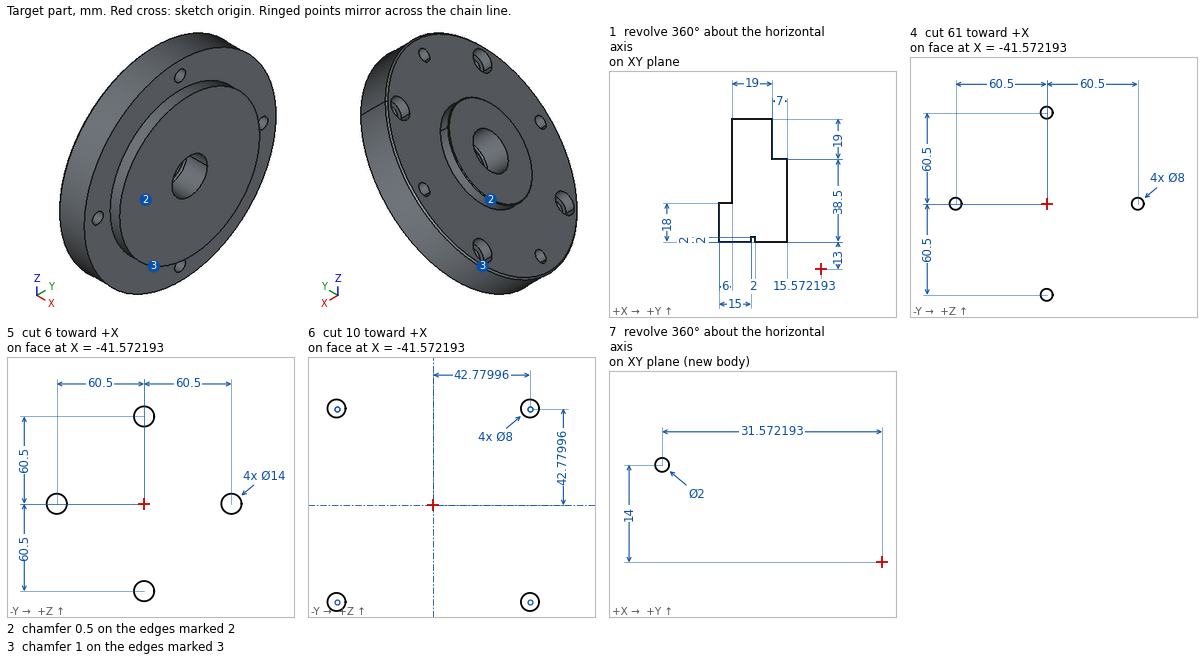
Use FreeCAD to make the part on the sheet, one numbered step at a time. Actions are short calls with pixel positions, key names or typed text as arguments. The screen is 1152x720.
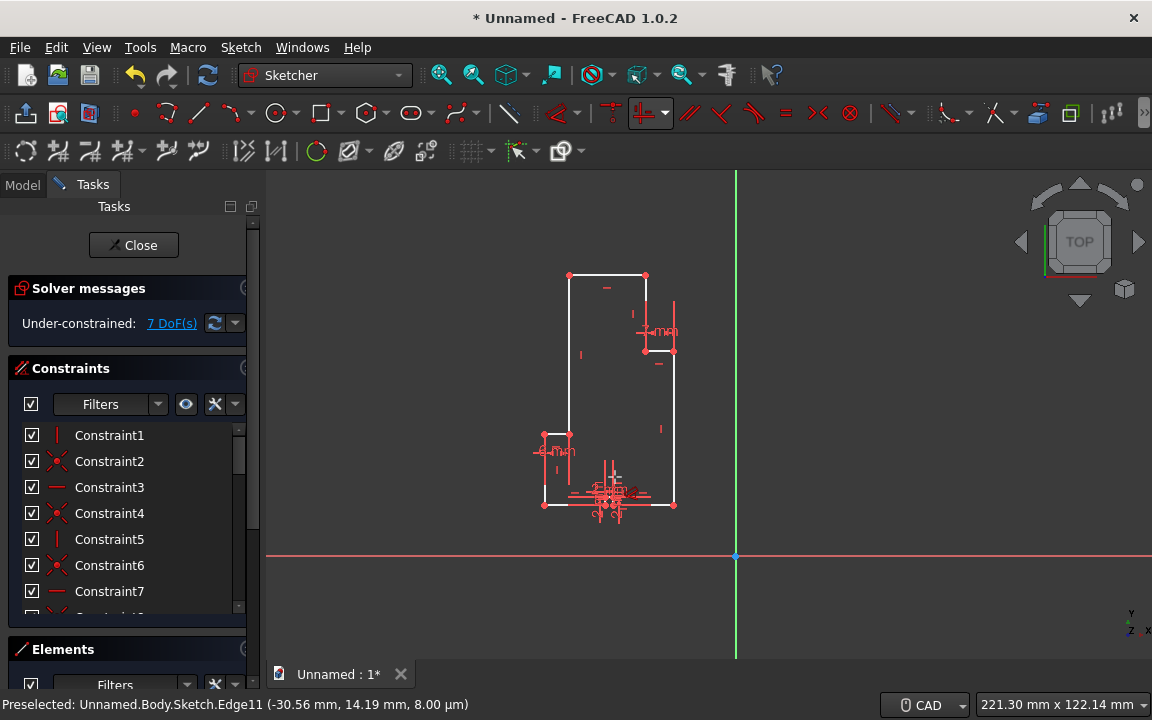
click(646, 328)
click(680, 296)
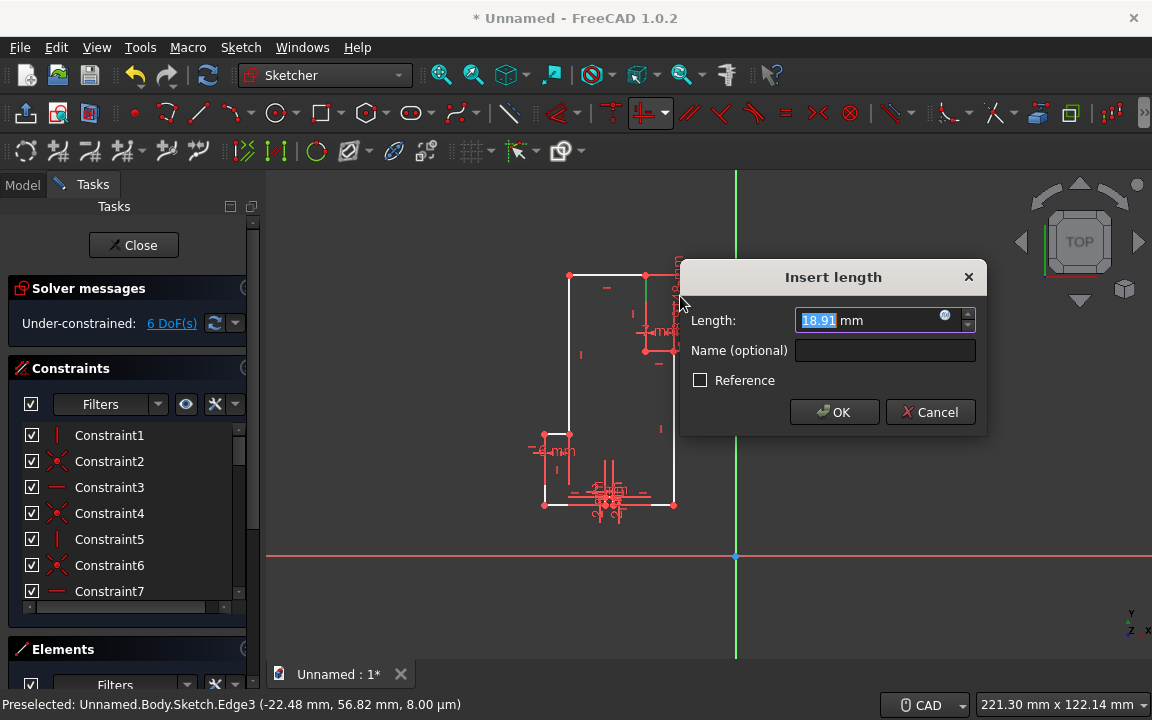
text(19)
key(Return)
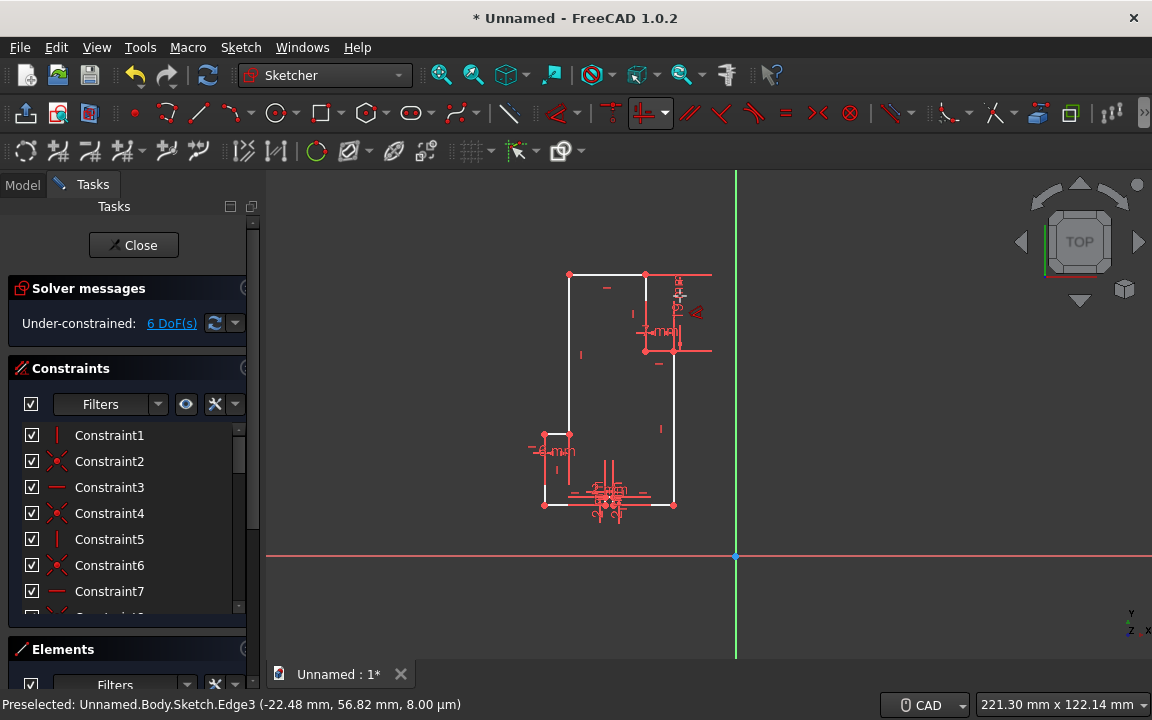
click(623, 275)
click(607, 241)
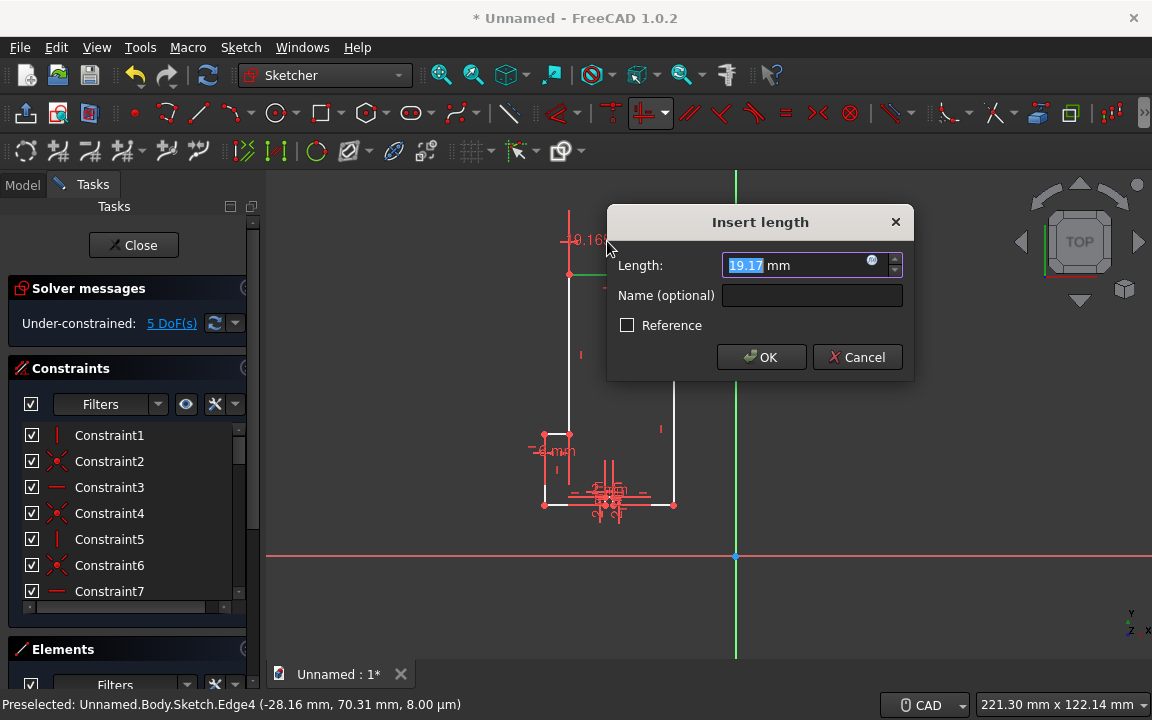
text(19)
key(Return)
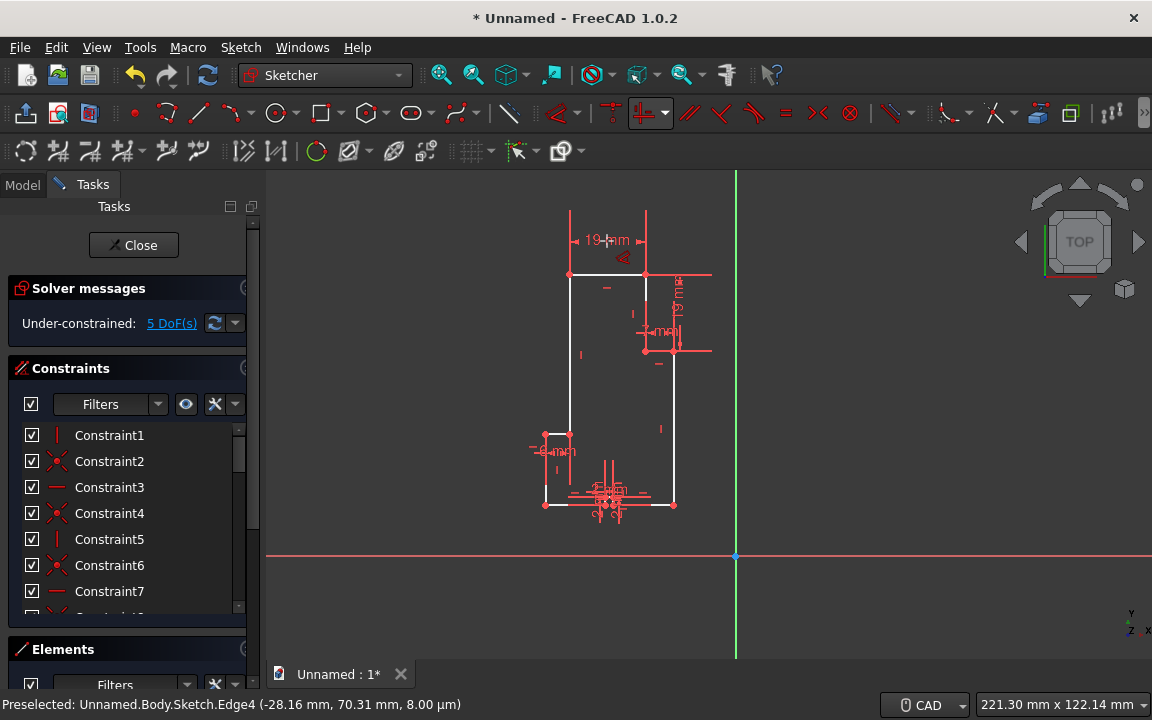
click(546, 455)
click(512, 486)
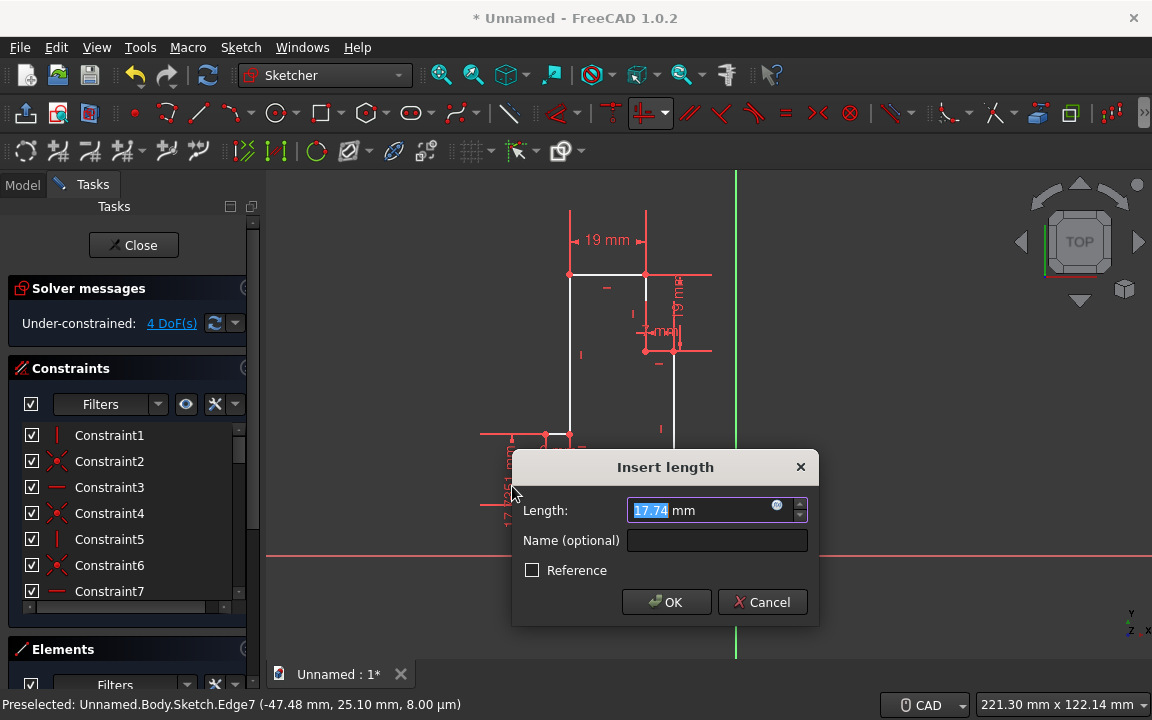
text(18)
key(Return)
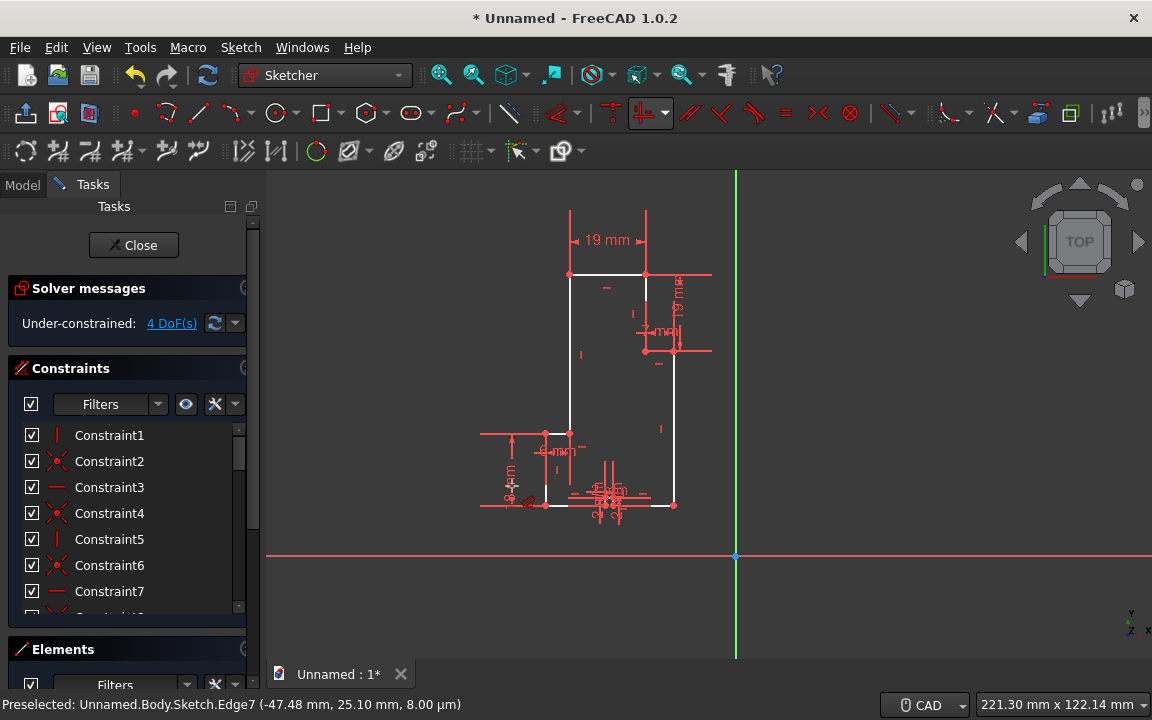
click(564, 506)
click(576, 540)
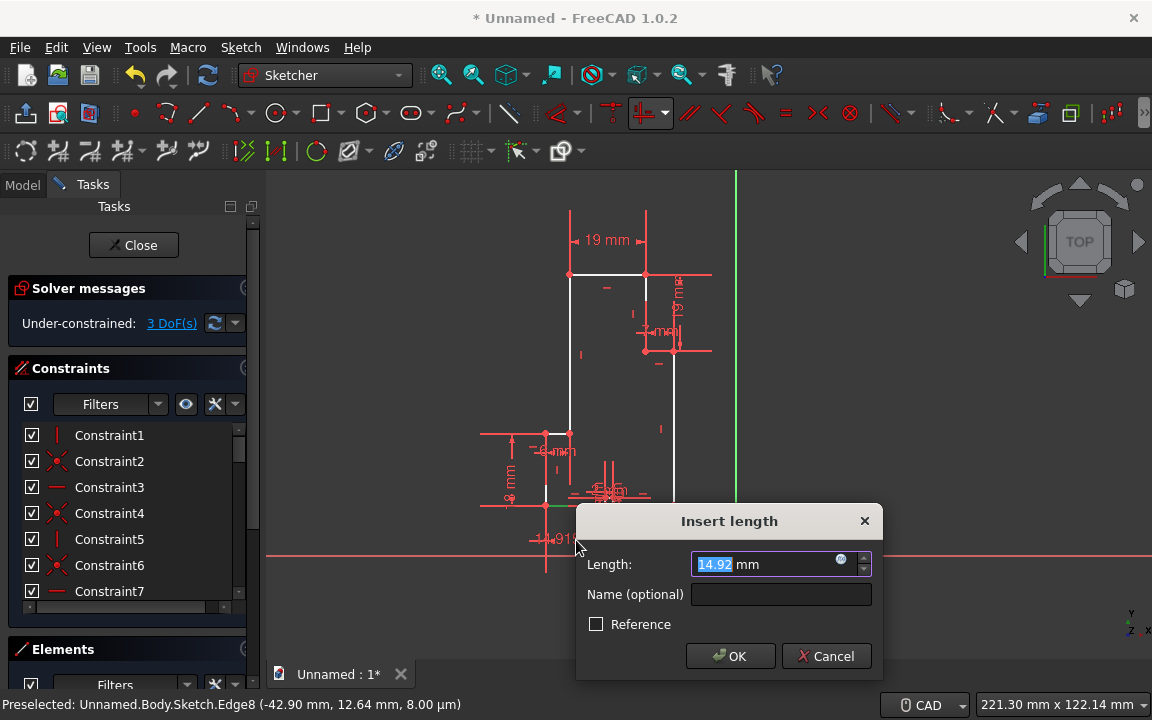
text(15)
key(Return)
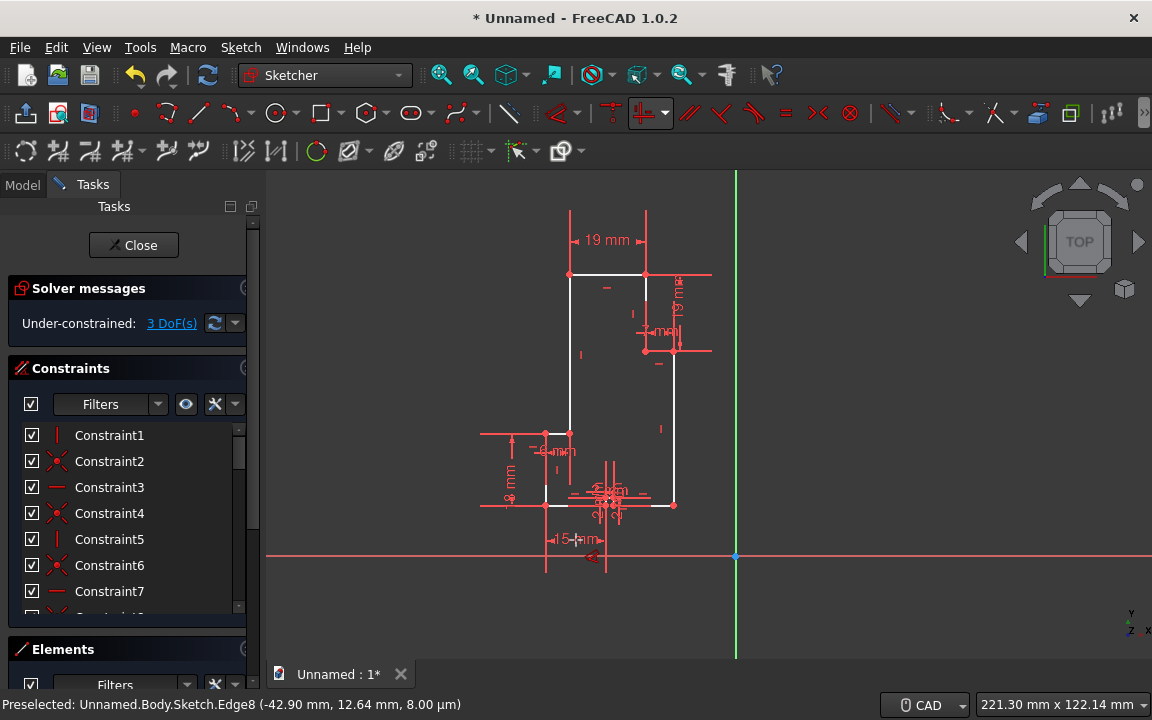
click(674, 506)
click(770, 531)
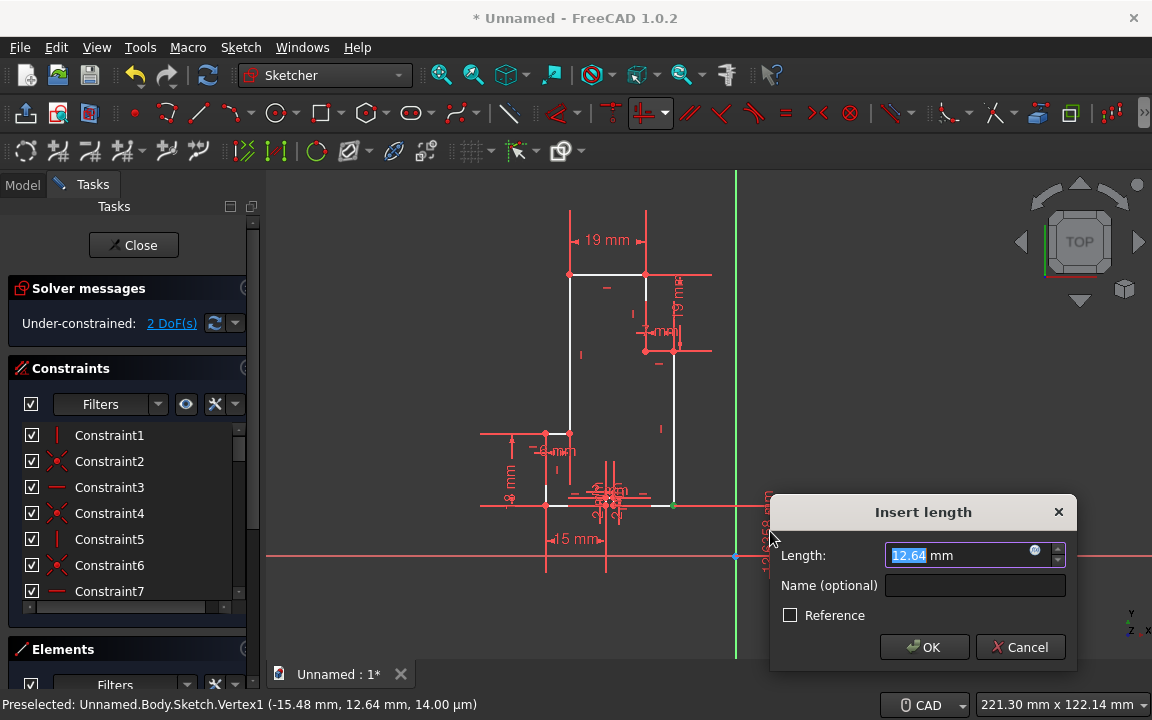
text(13)
key(Return)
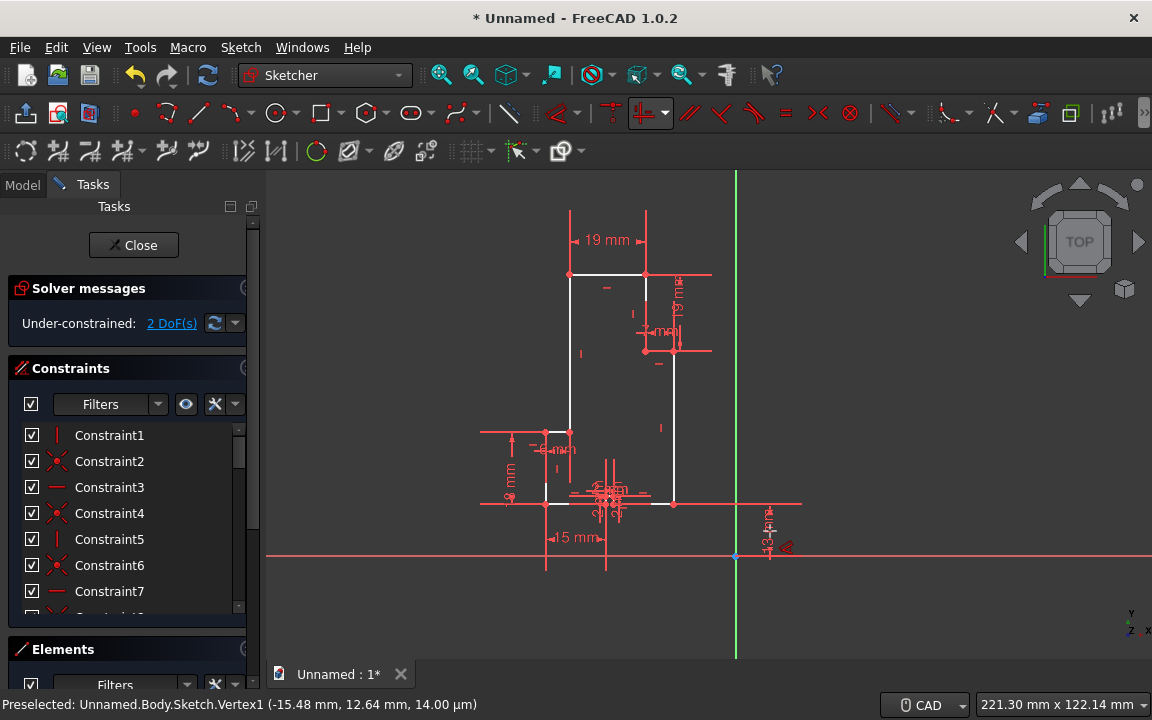
click(674, 458)
click(708, 428)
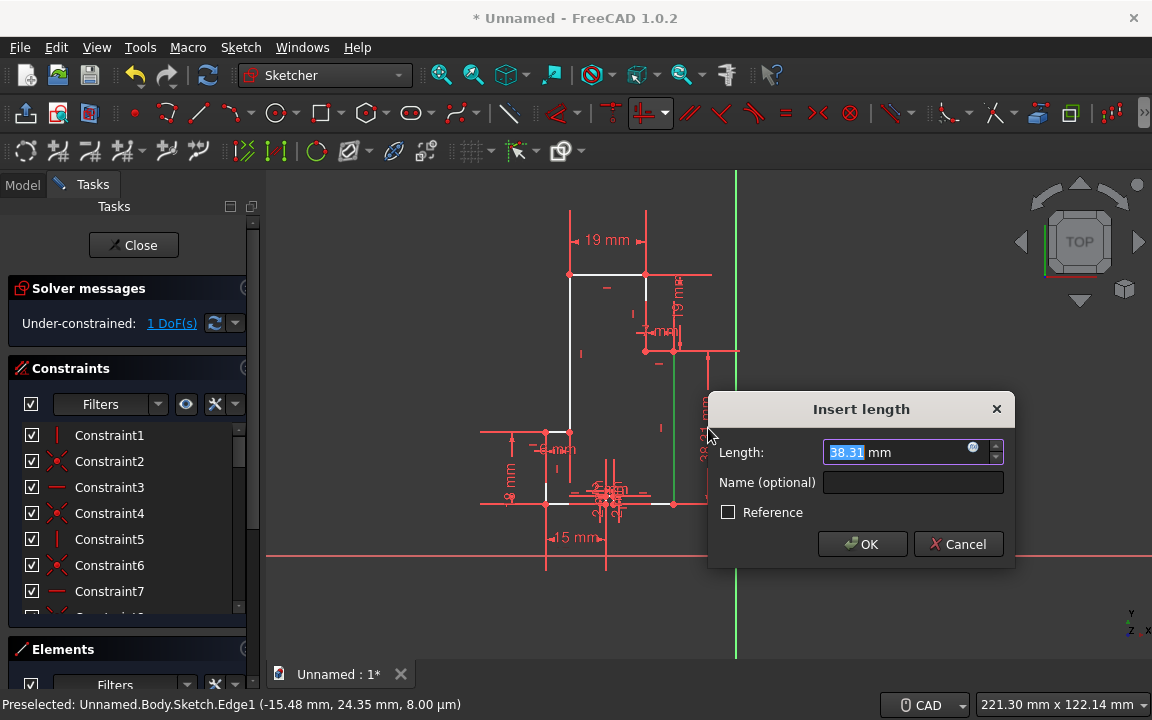
text(38.5)
key(Return)